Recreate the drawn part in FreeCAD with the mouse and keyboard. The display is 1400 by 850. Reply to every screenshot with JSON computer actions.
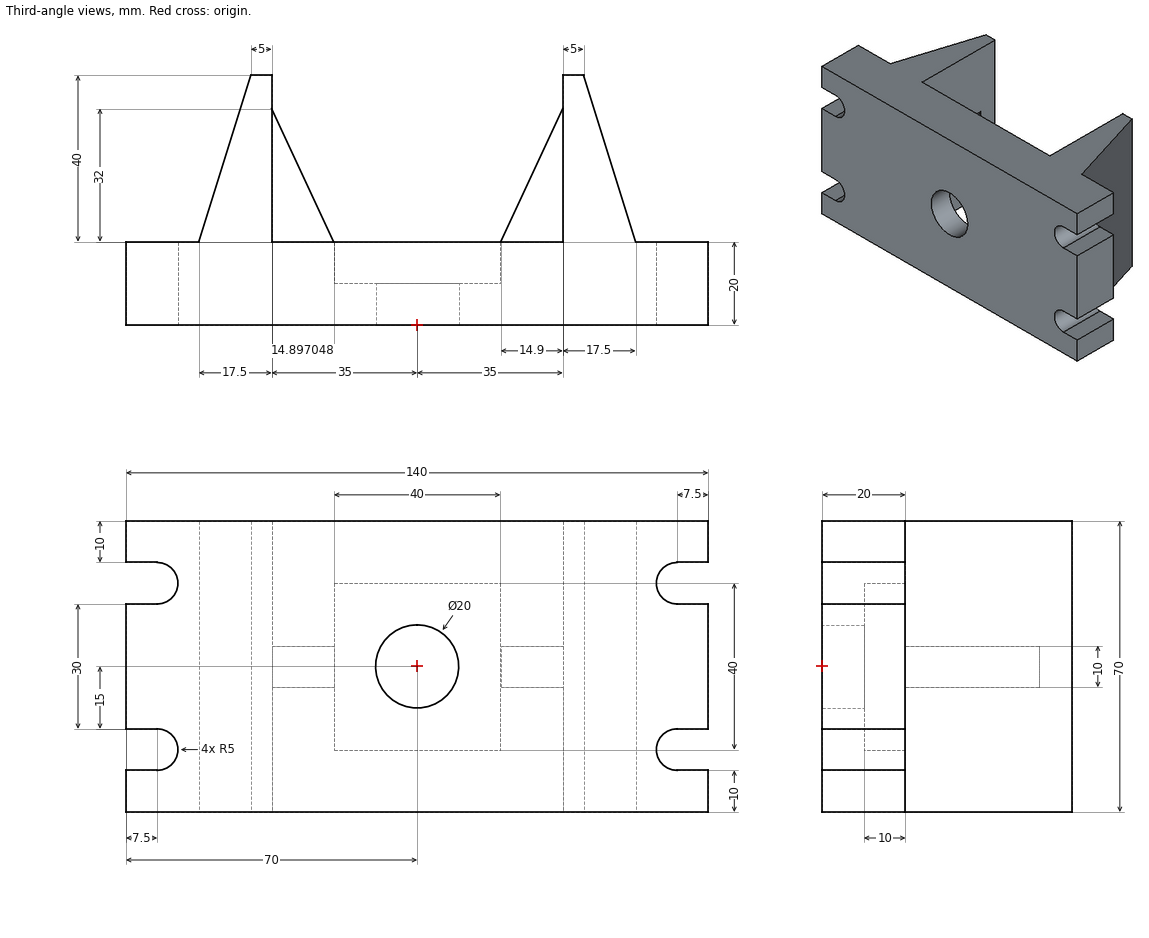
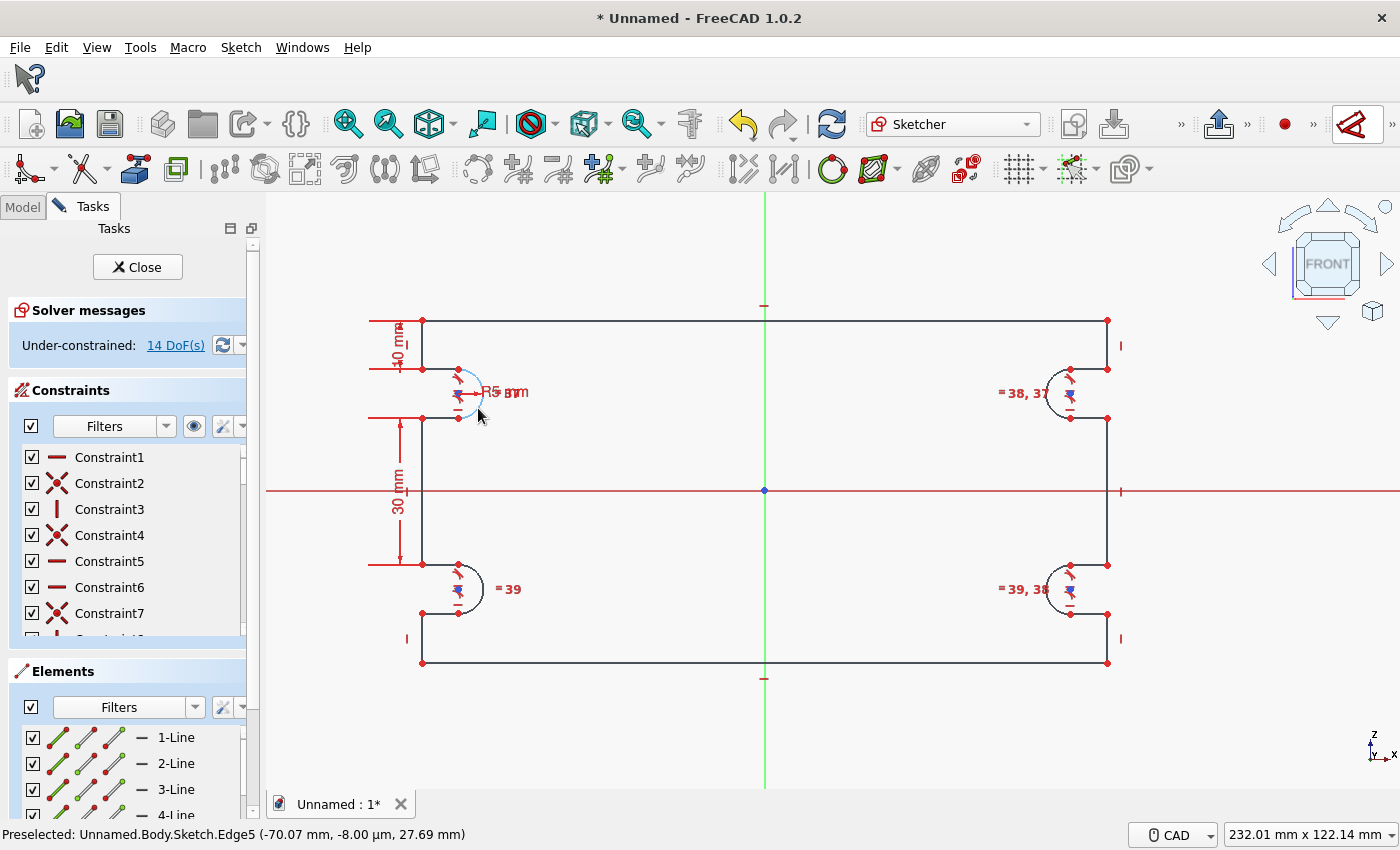
{"action": "left_click", "coordinate": [1107, 335]}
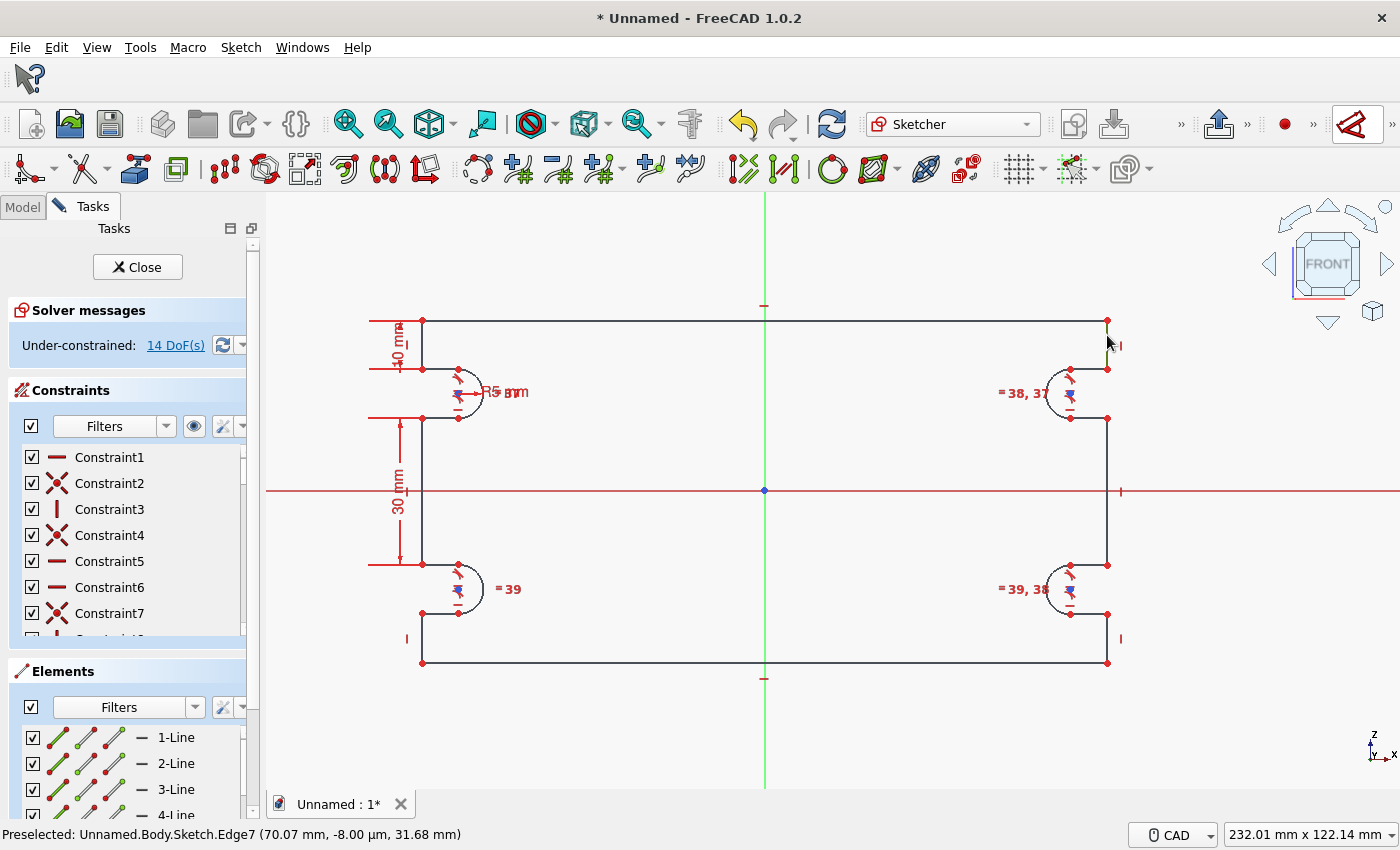
{"action": "key", "text": "i"}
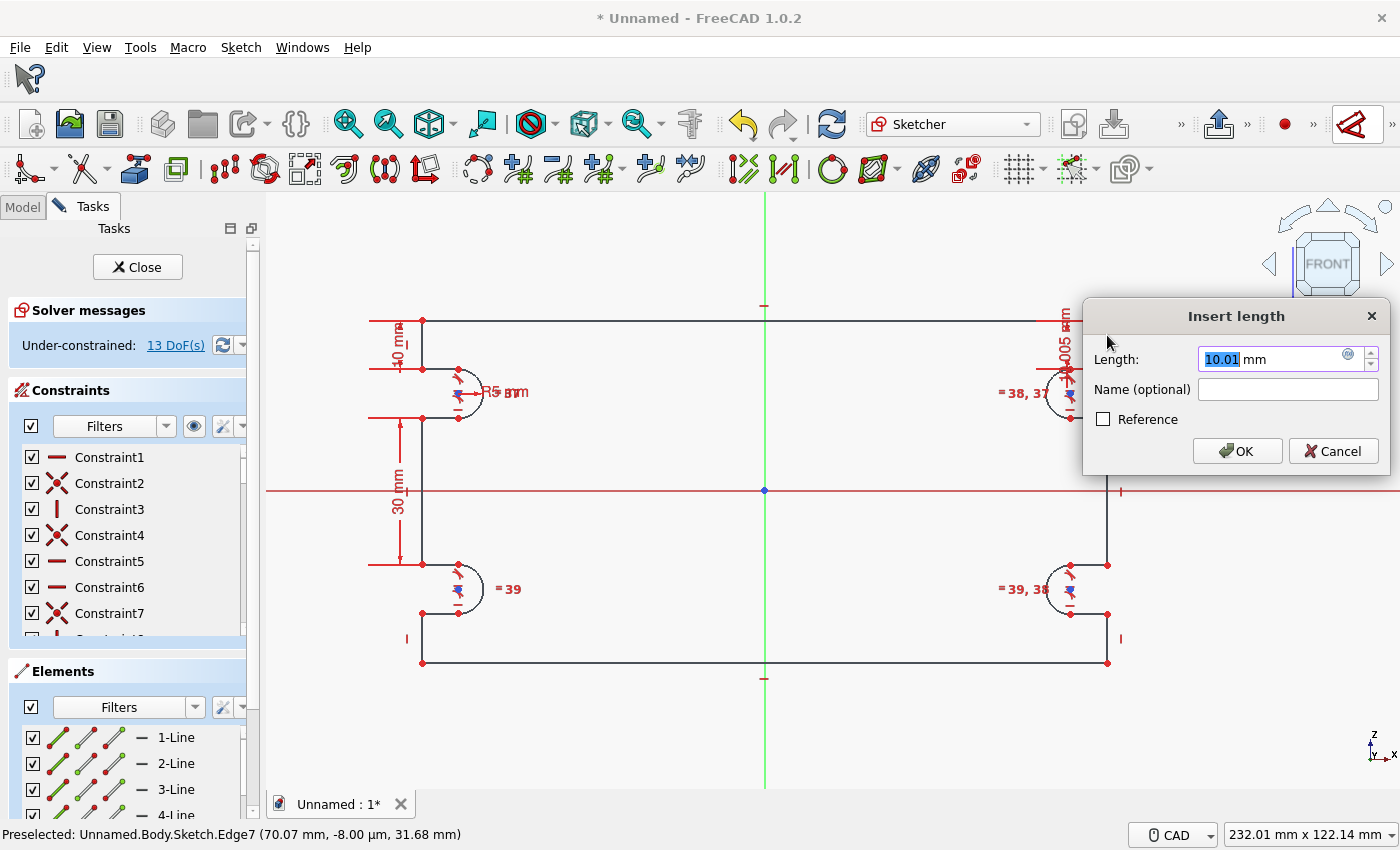
{"action": "type", "text": "10"}
{"action": "key", "text": "Return"}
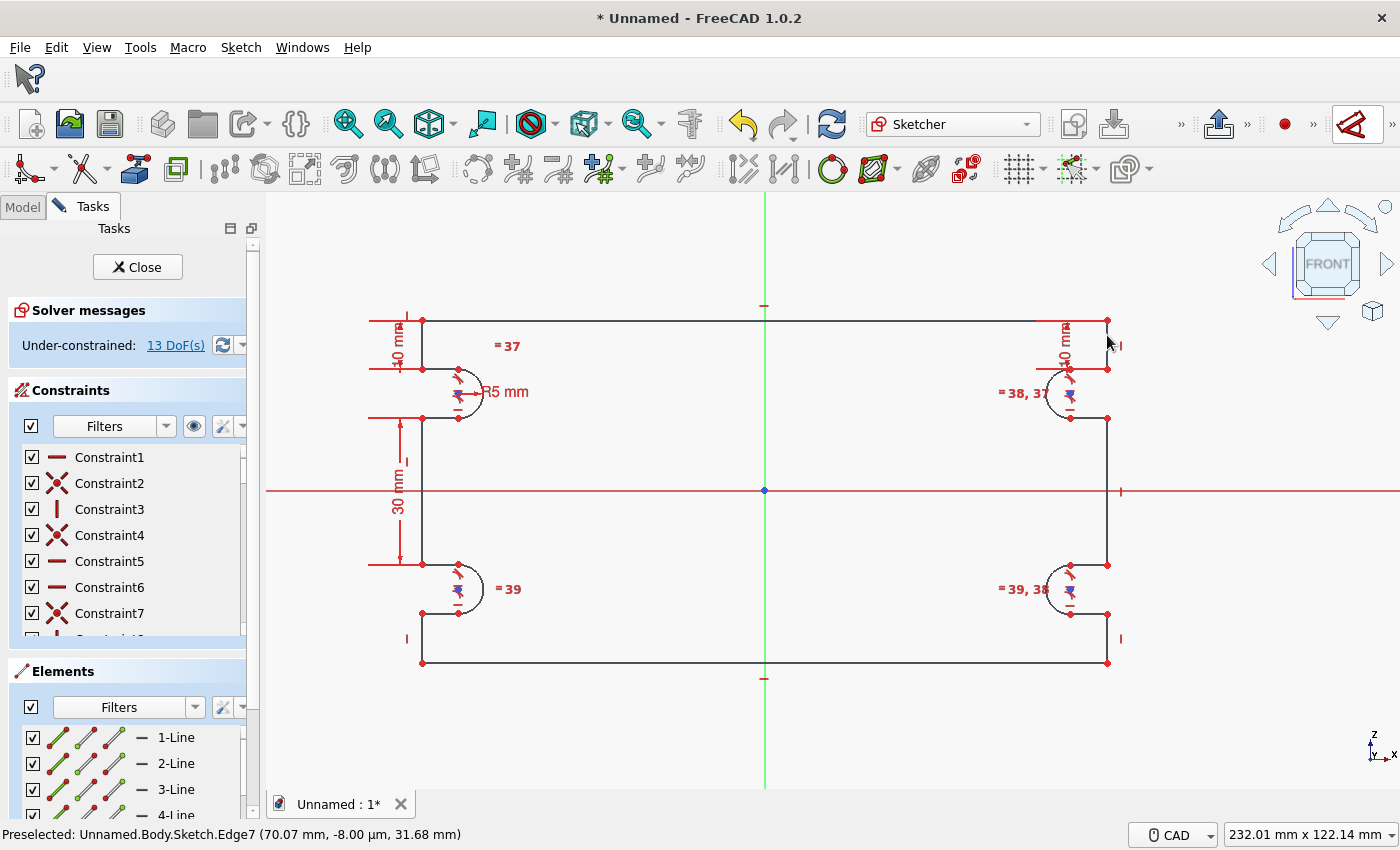
{"action": "left_click", "coordinate": [1107, 462]}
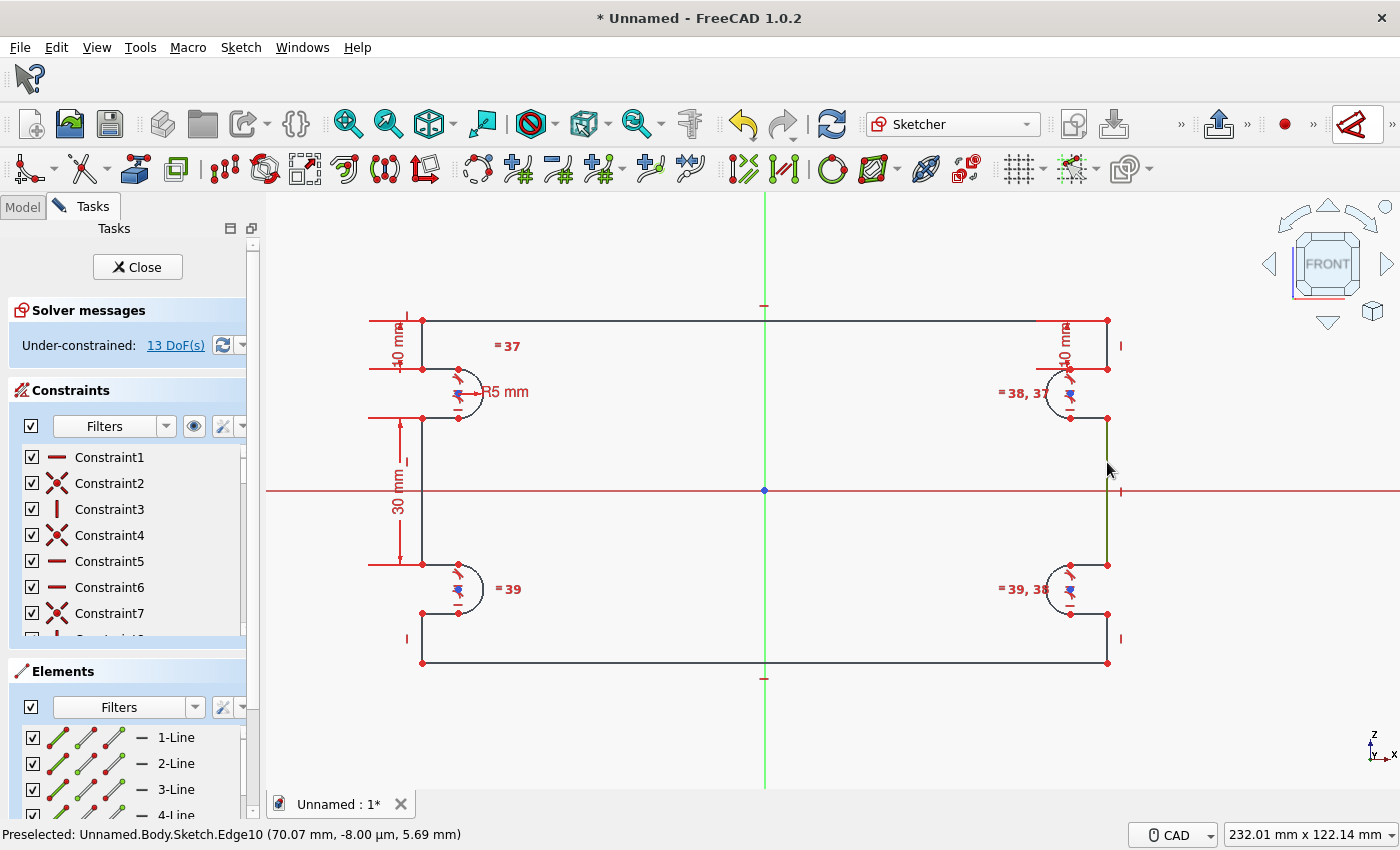
{"action": "left_click", "coordinate": [1378, 124]}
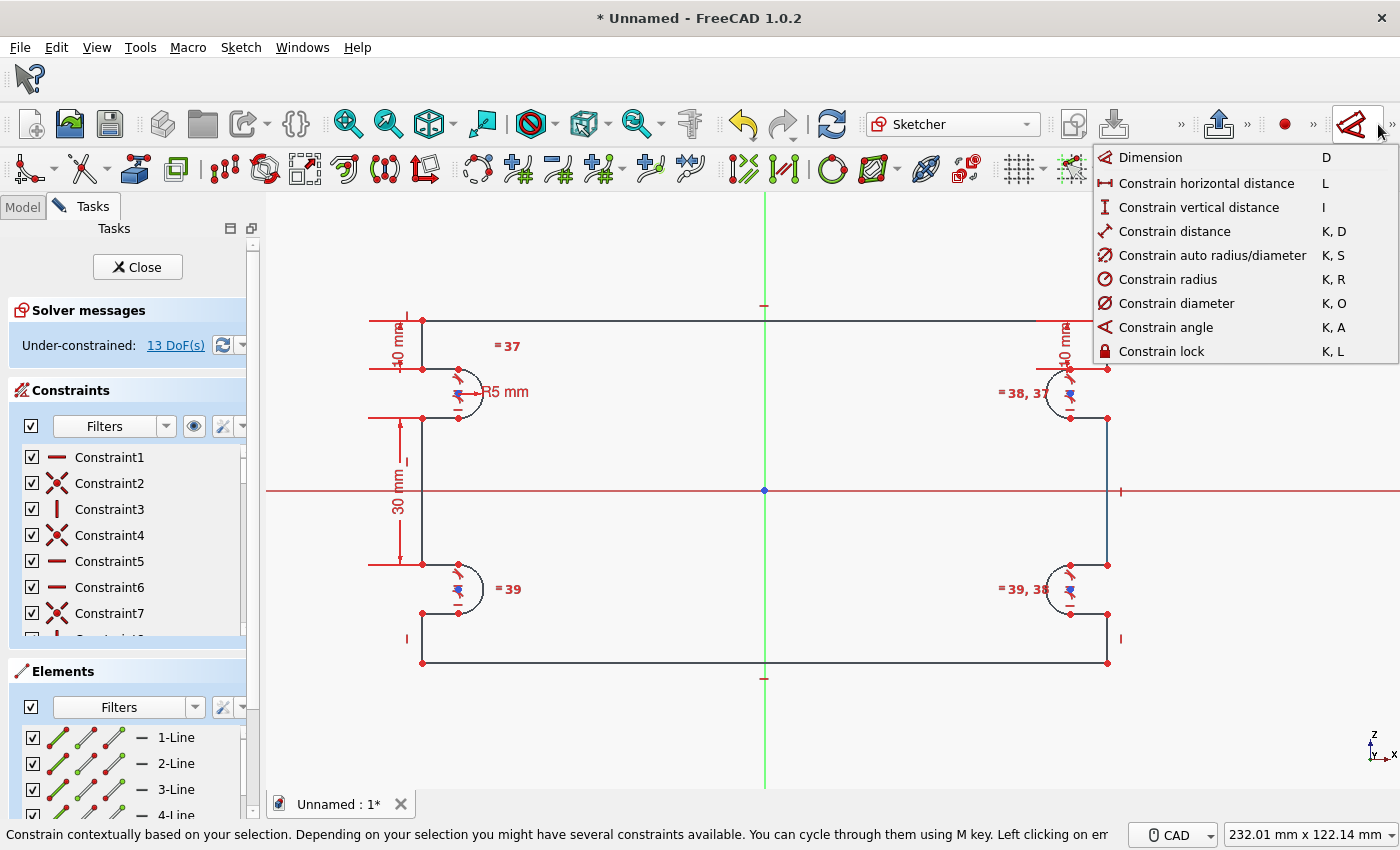
{"action": "left_click", "coordinate": [1246, 207]}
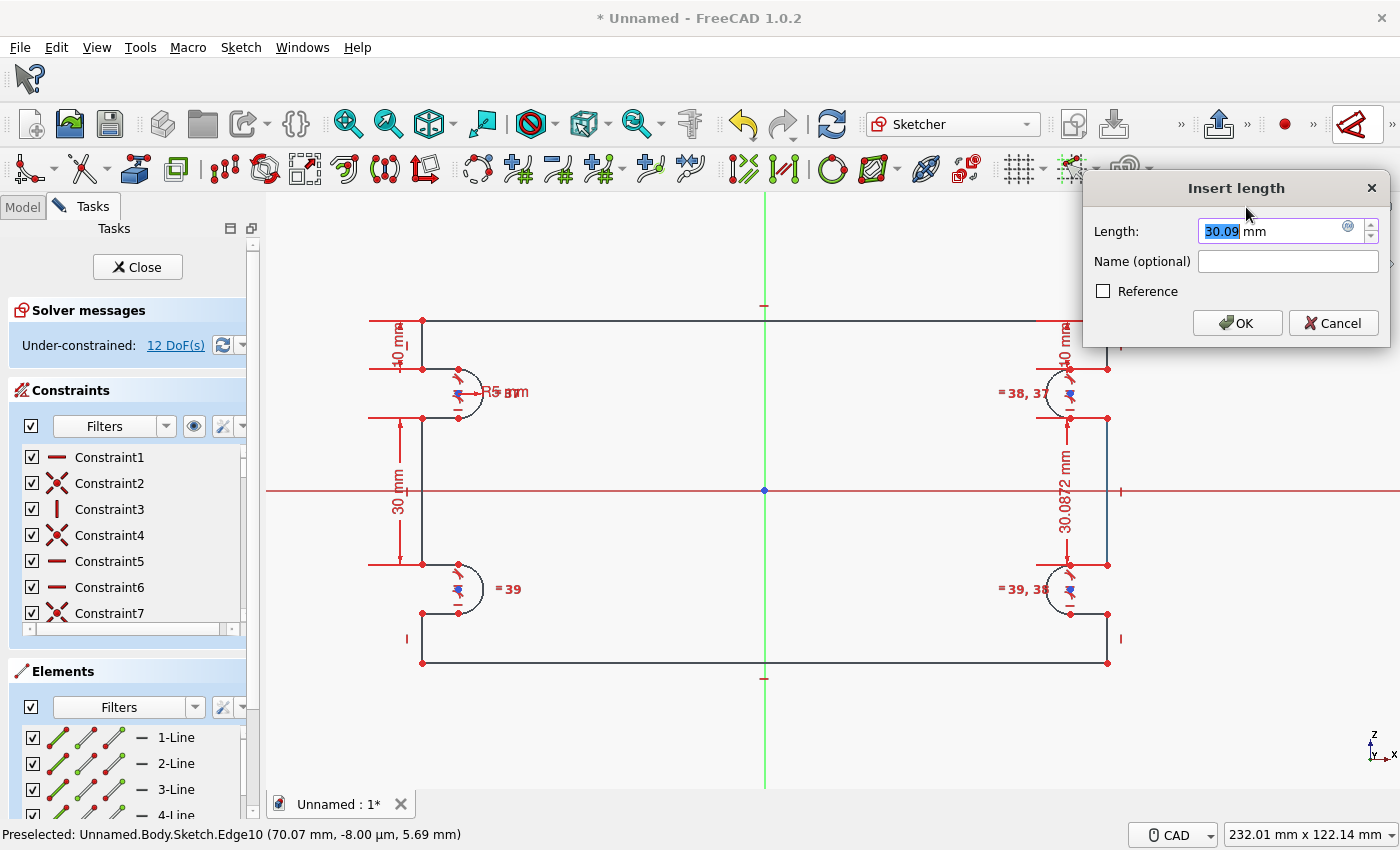
{"action": "type", "text": "30"}
{"action": "key", "text": "Return"}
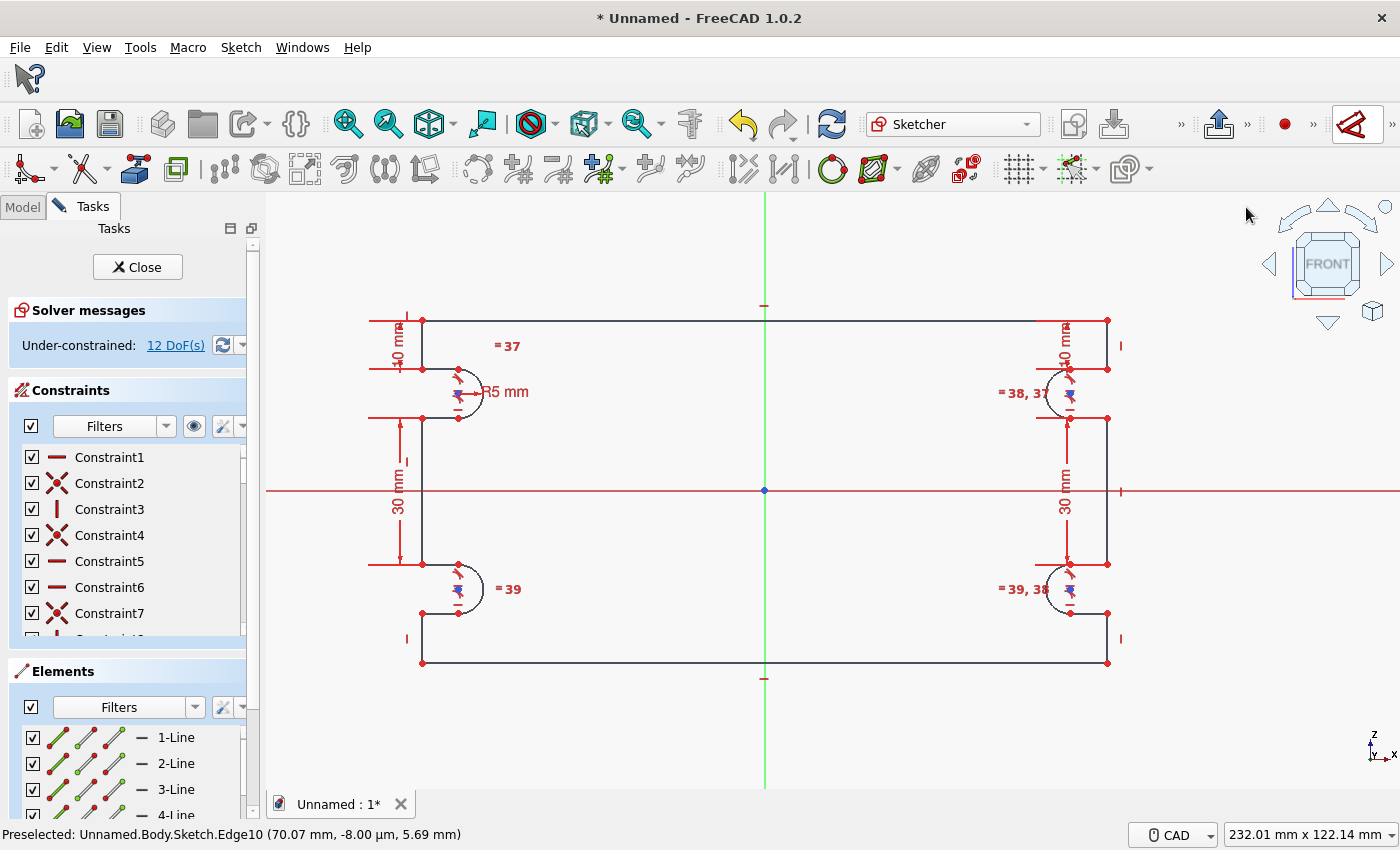
{"action": "left_click", "coordinate": [1107, 629]}